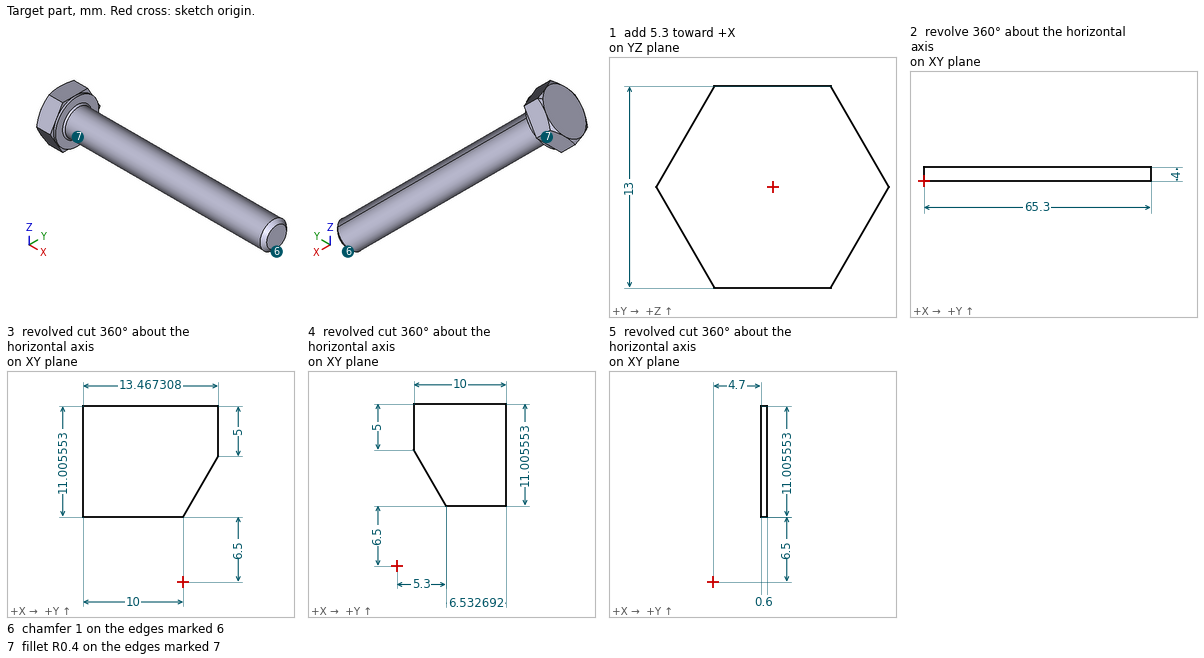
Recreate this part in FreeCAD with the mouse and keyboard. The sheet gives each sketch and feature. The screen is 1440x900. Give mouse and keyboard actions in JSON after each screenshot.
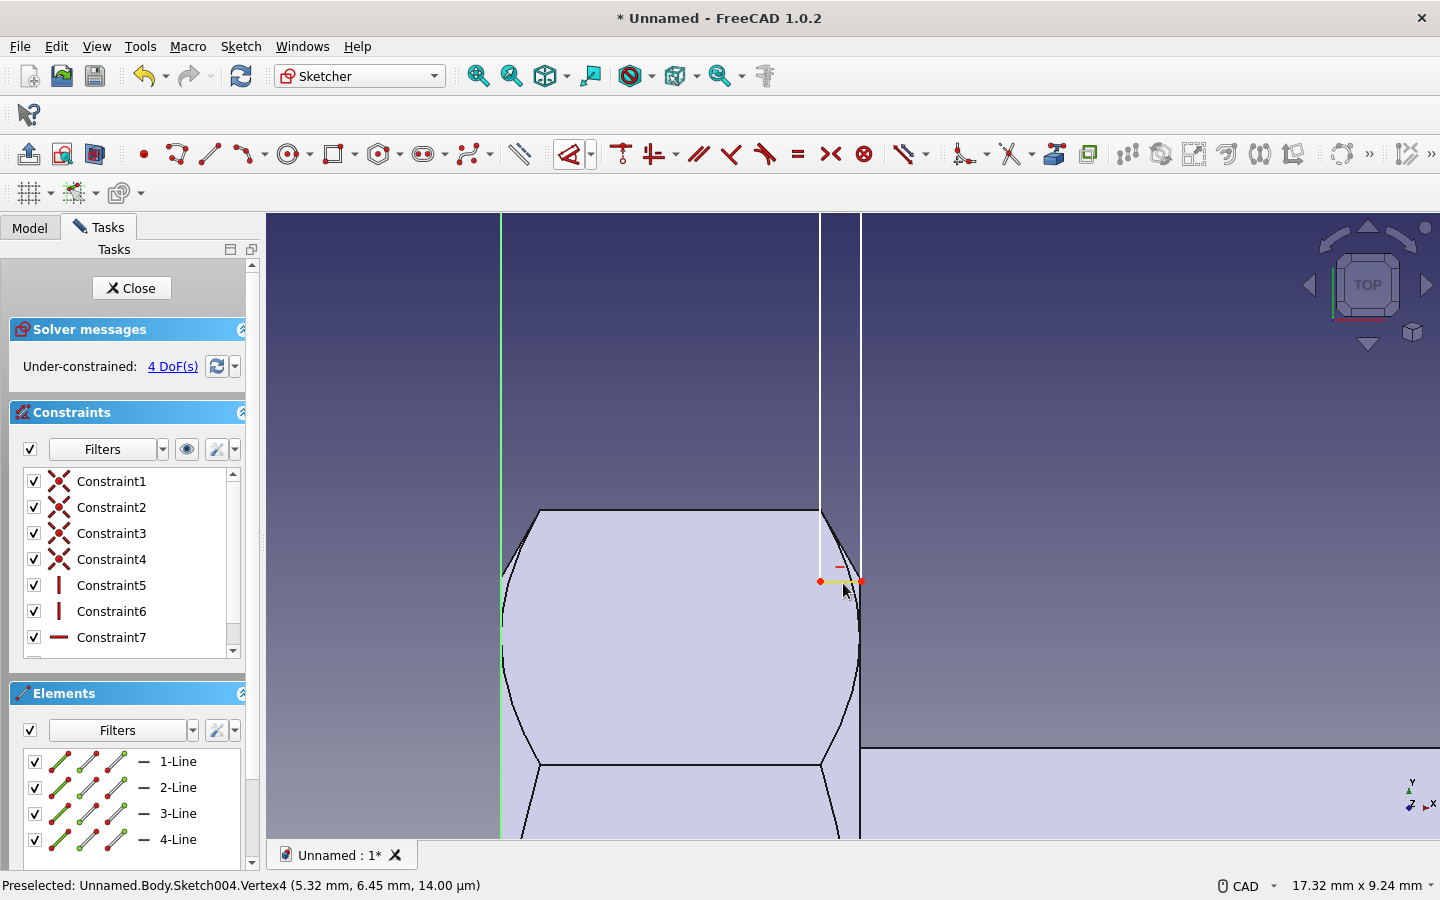
{"action": "left_click", "coordinate": [841, 582]}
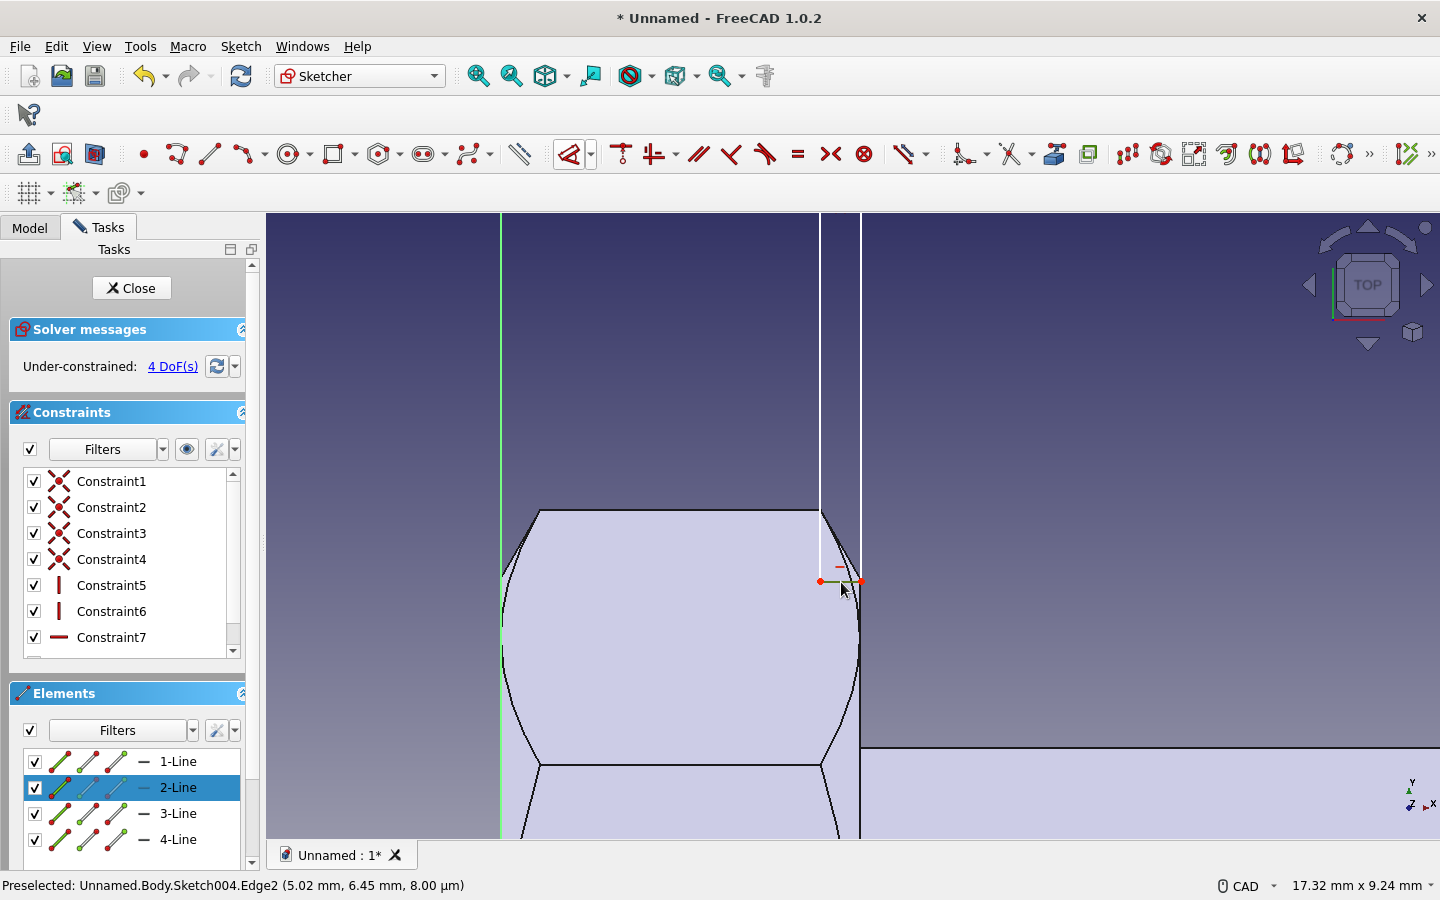
{"action": "left_click", "coordinate": [590, 154]}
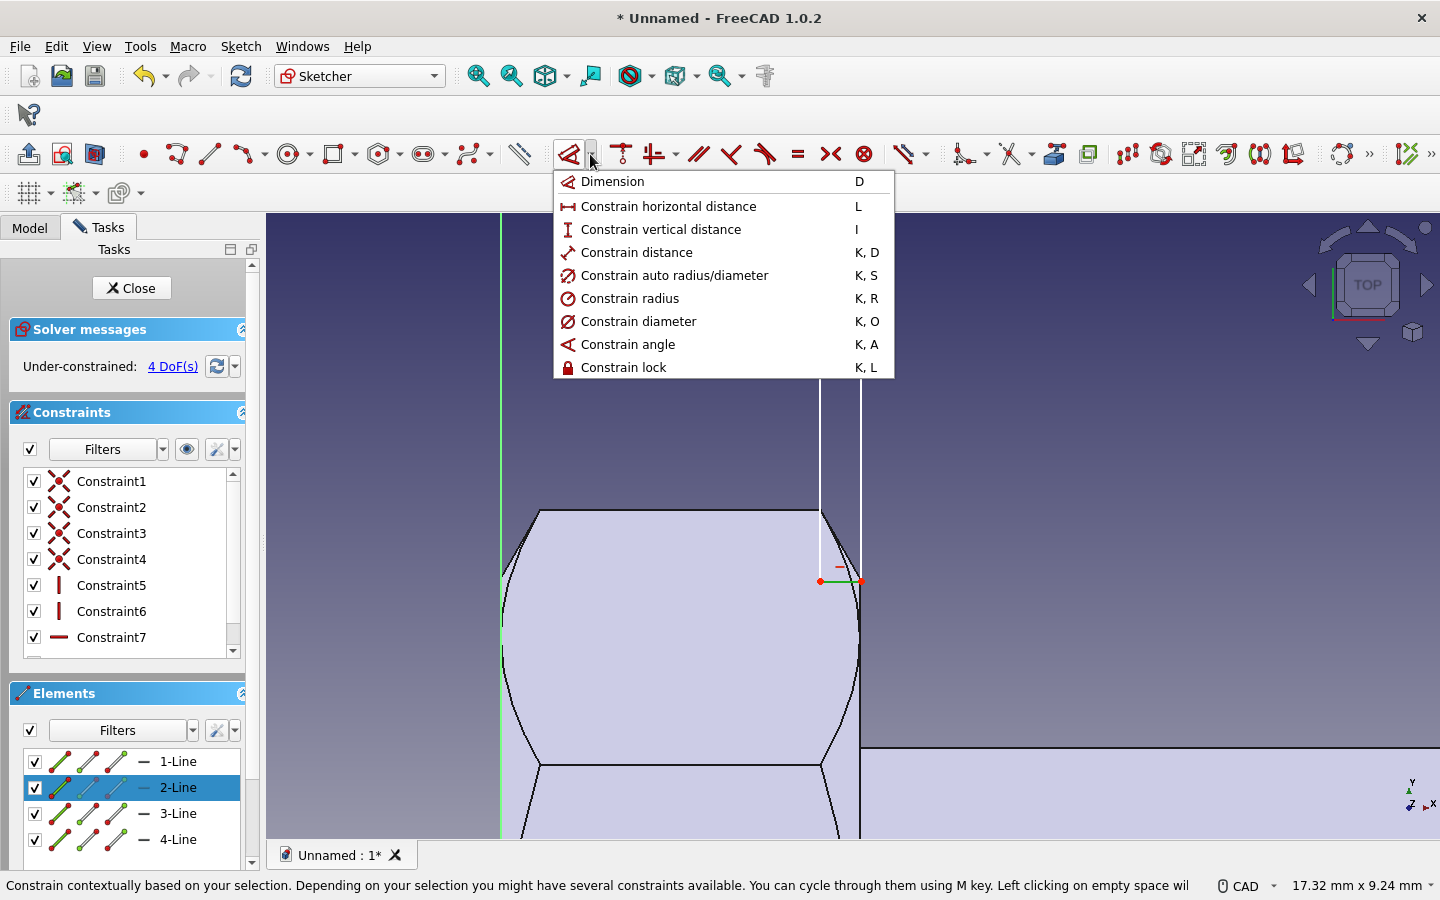
{"action": "left_click", "coordinate": [724, 206]}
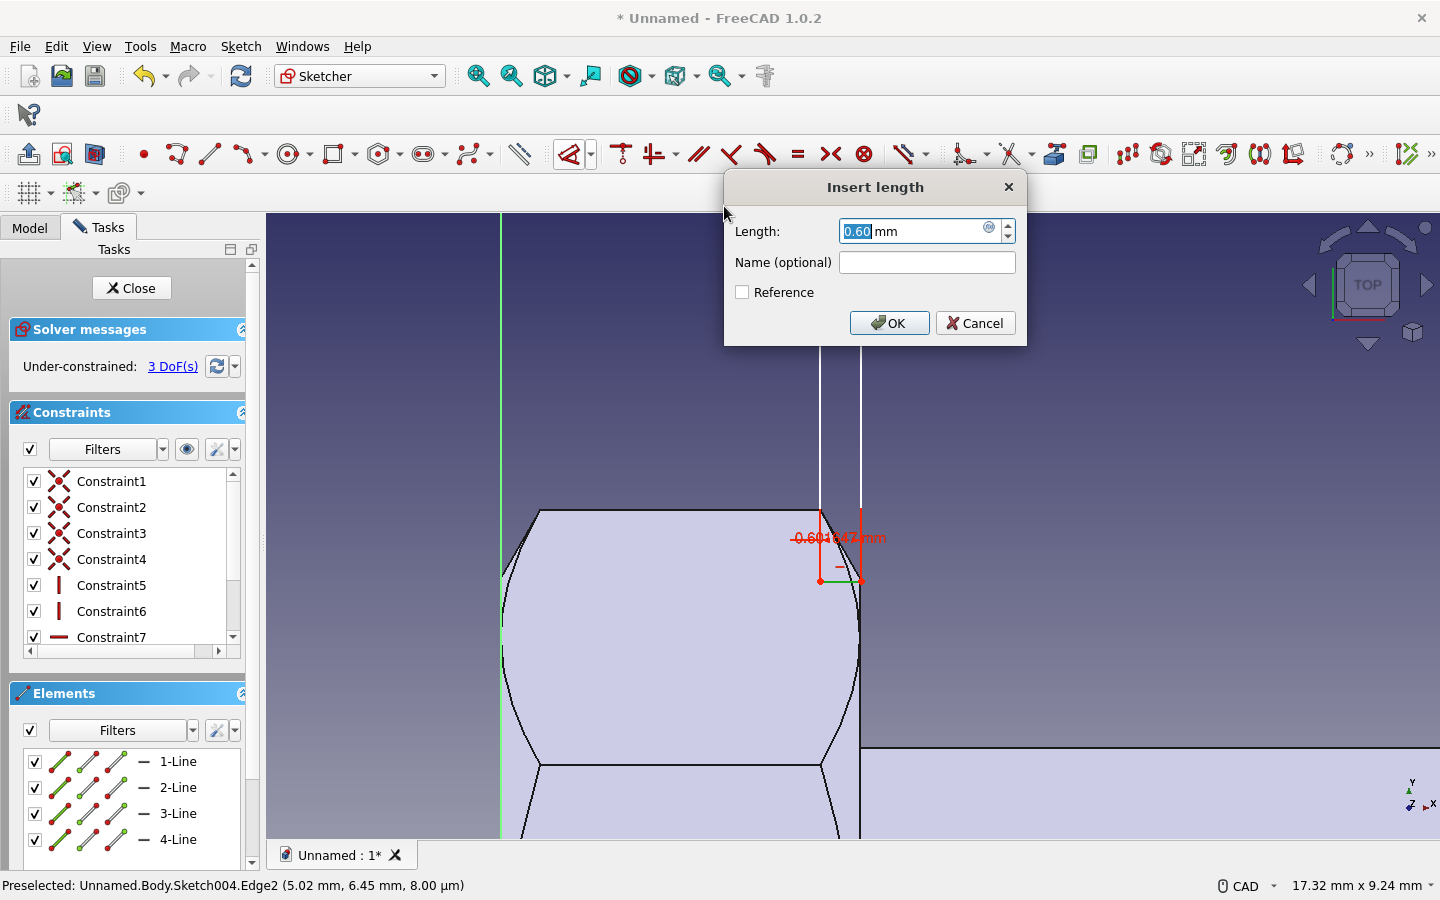
{"action": "type", "text": "0.6"}
{"action": "key", "text": "Return"}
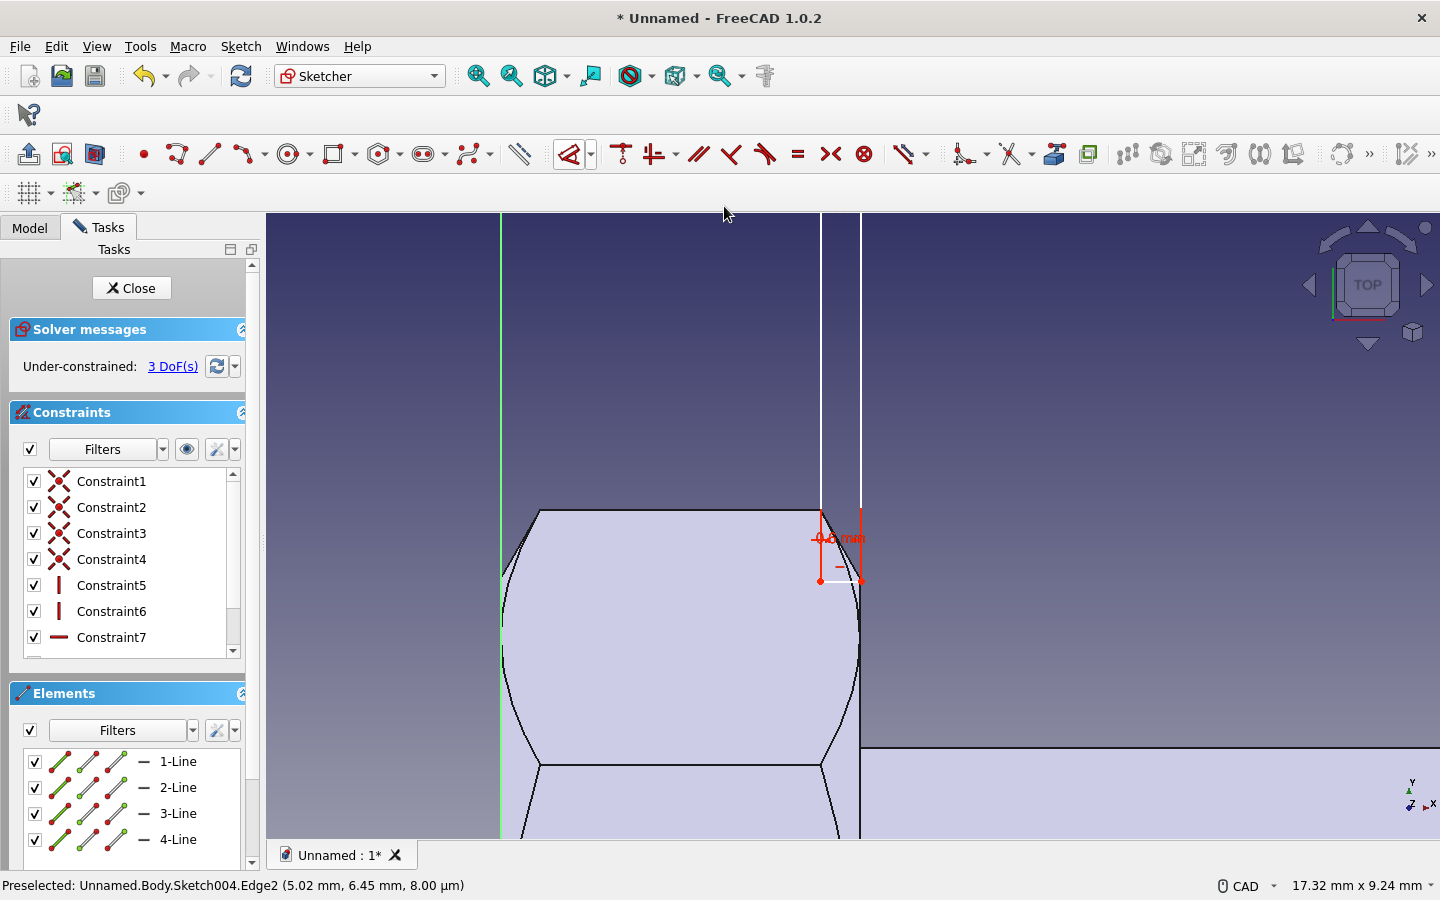
{"action": "scroll", "coordinate": [845, 584], "scroll_direction": "down", "scroll_amount": 5}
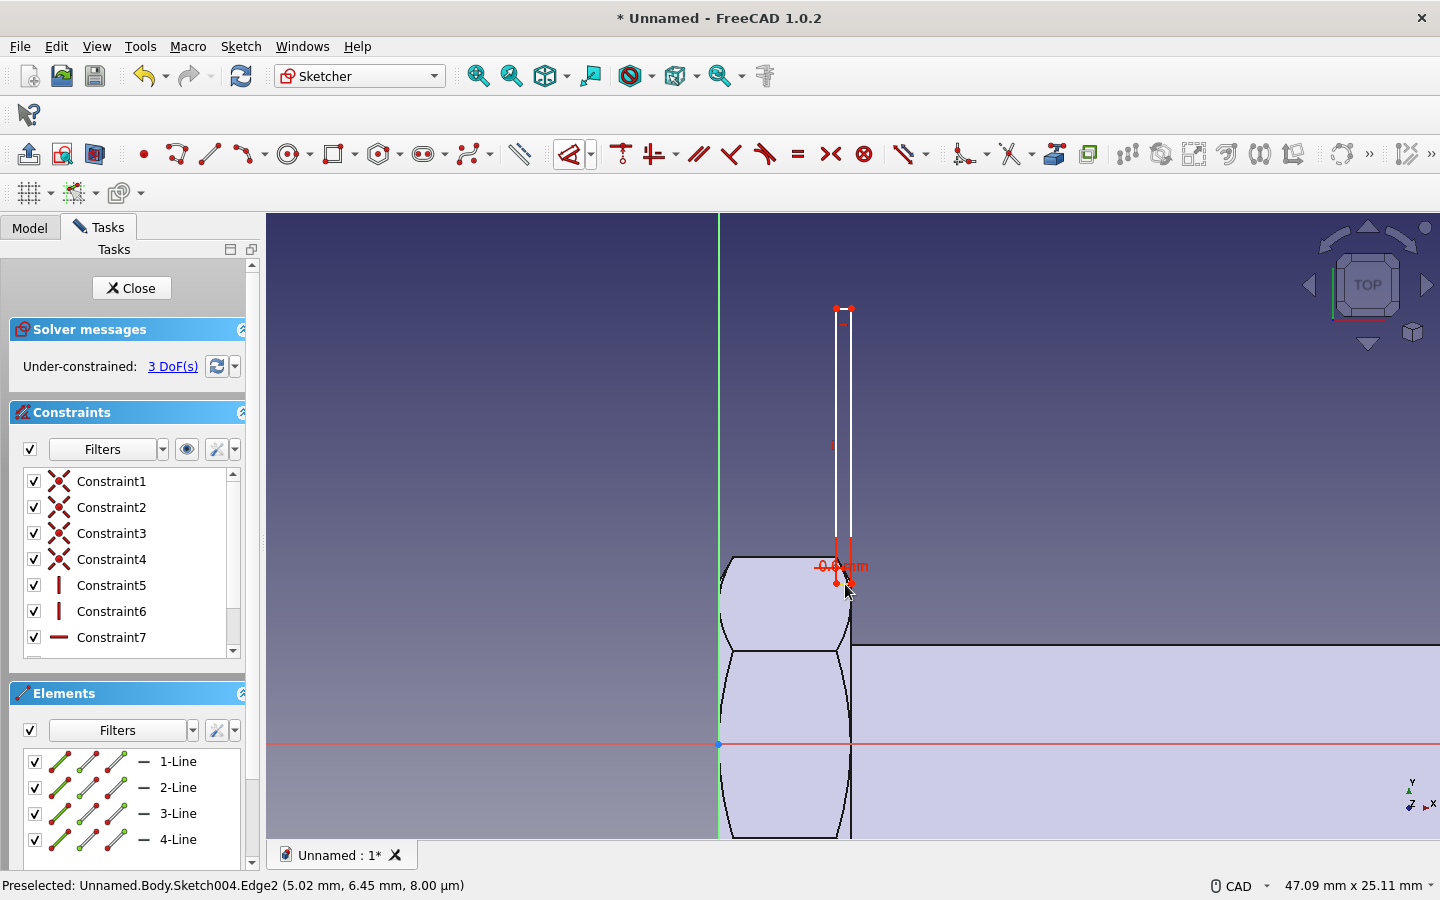
{"action": "left_click", "coordinate": [836, 309]}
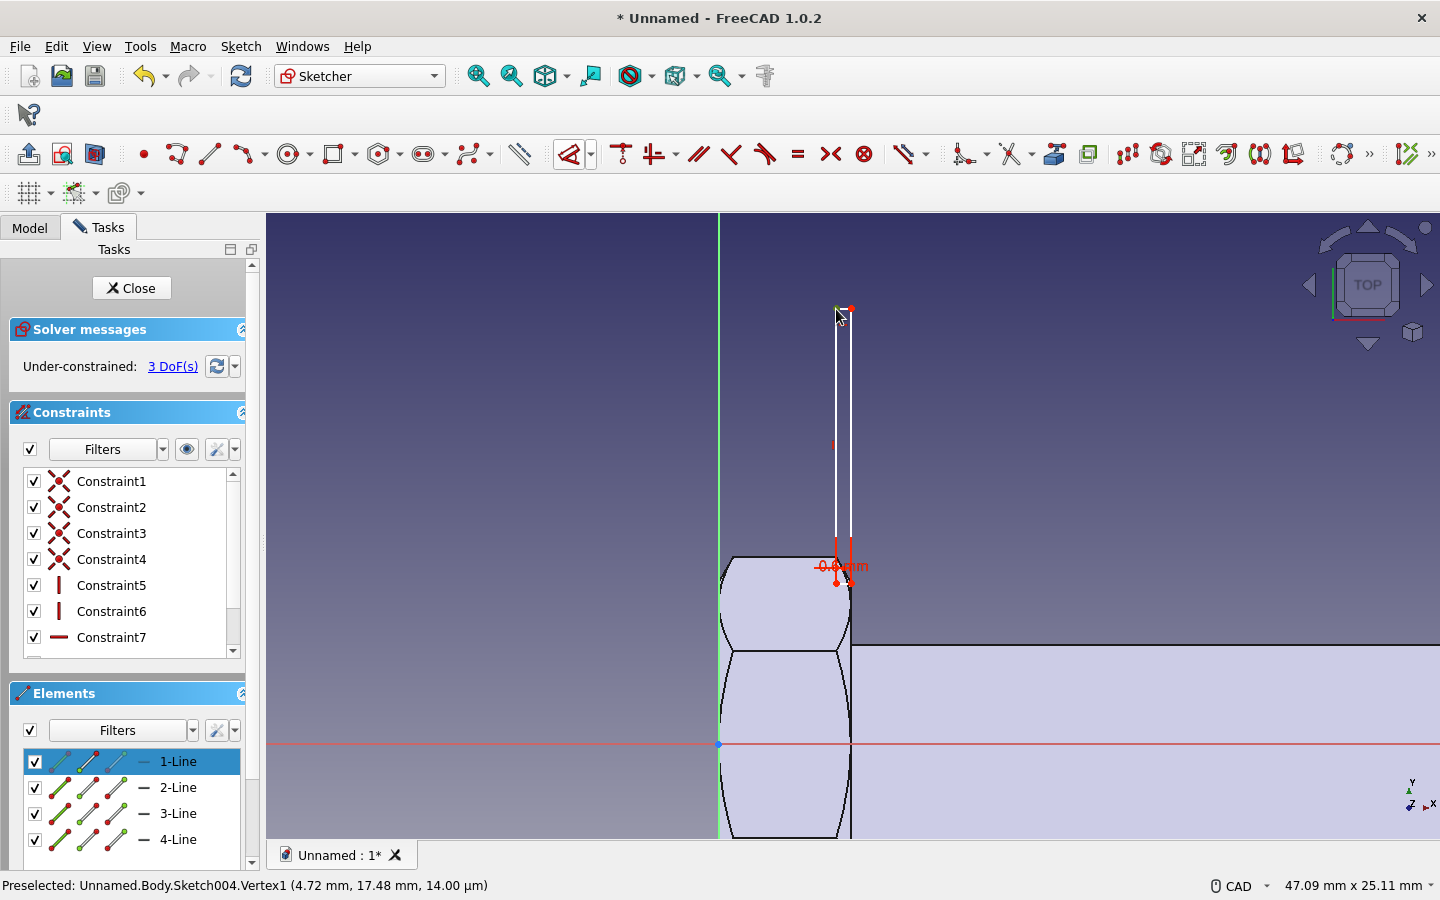
{"action": "key", "text": "l"}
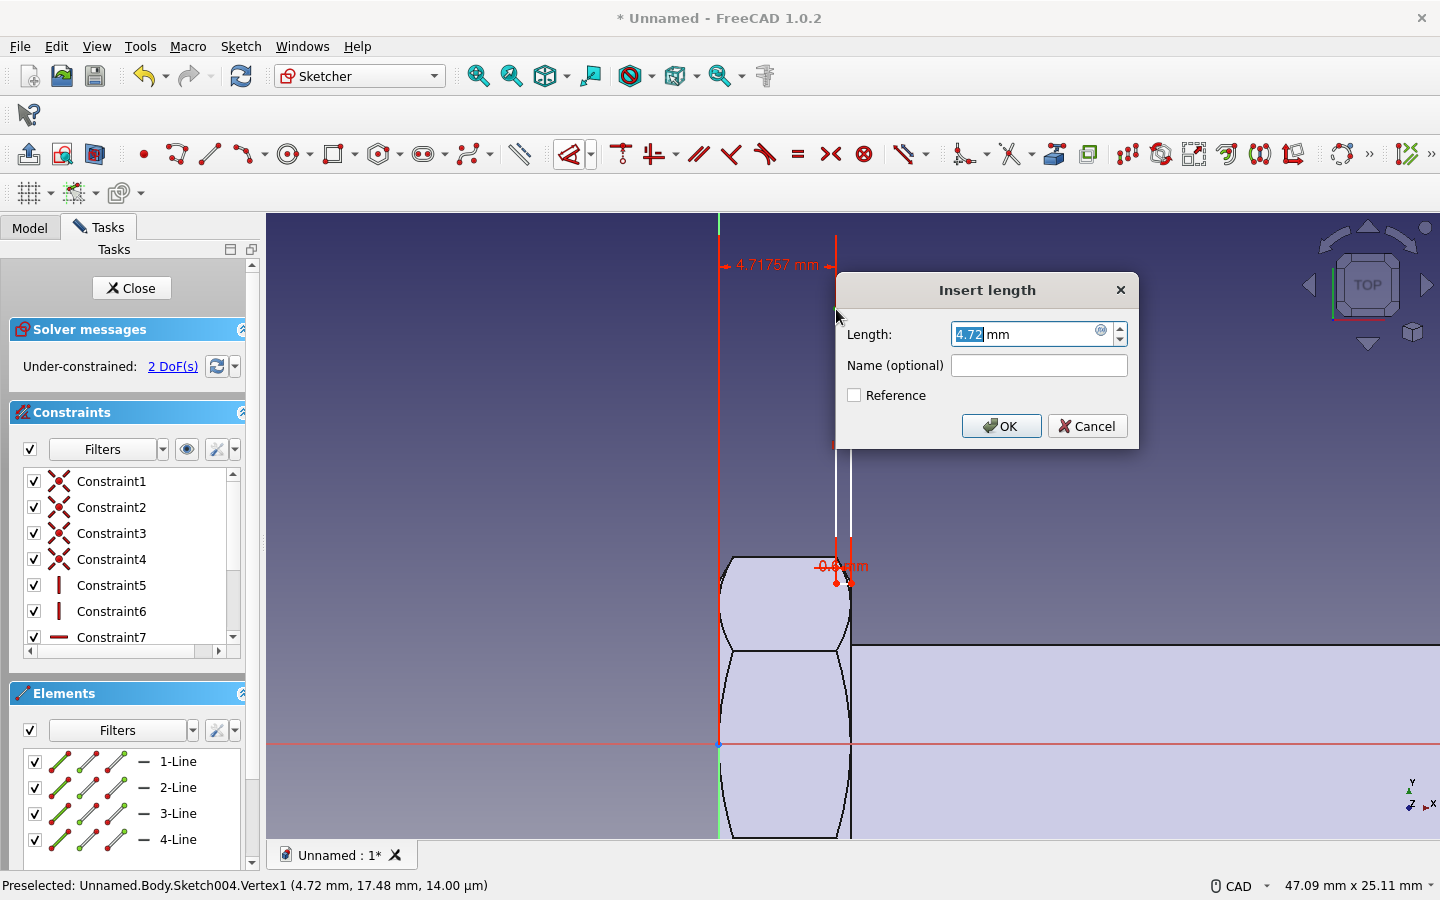
{"action": "type", "text": "4.7"}
{"action": "key", "text": "Return"}